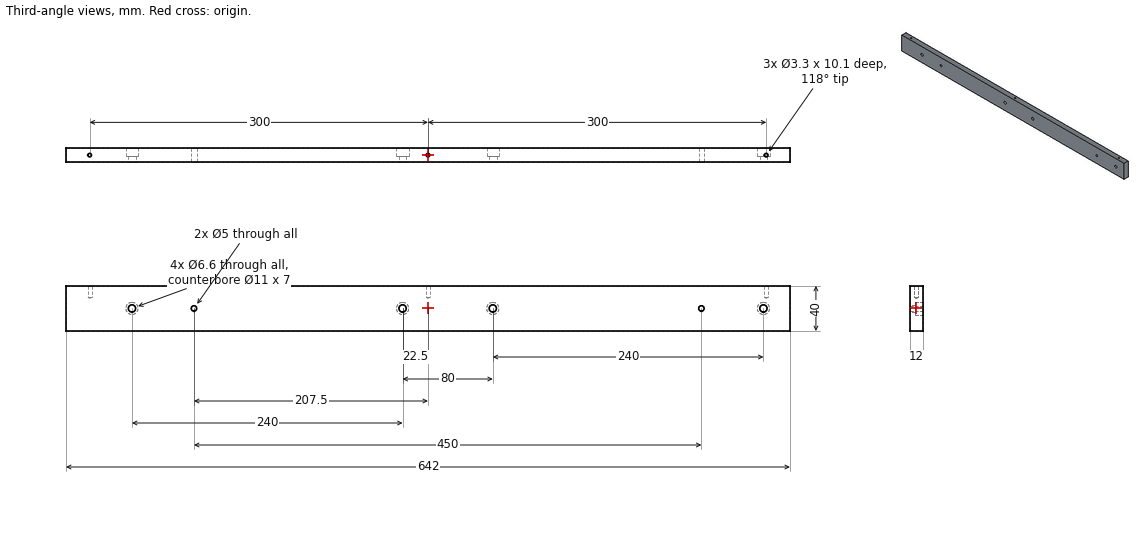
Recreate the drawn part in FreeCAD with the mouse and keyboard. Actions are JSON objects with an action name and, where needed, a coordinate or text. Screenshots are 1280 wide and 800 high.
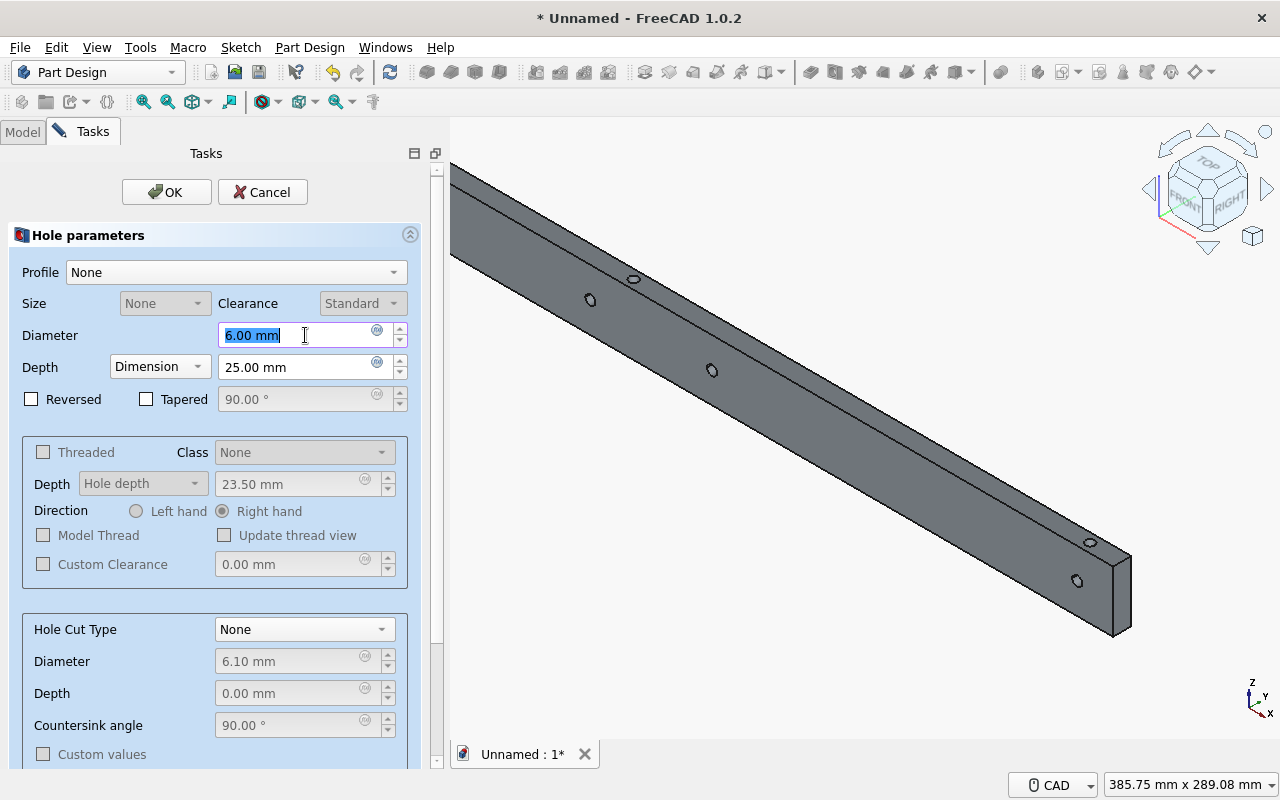
{"action": "type", "text": "3.3"}
{"action": "key", "text": "Tab"}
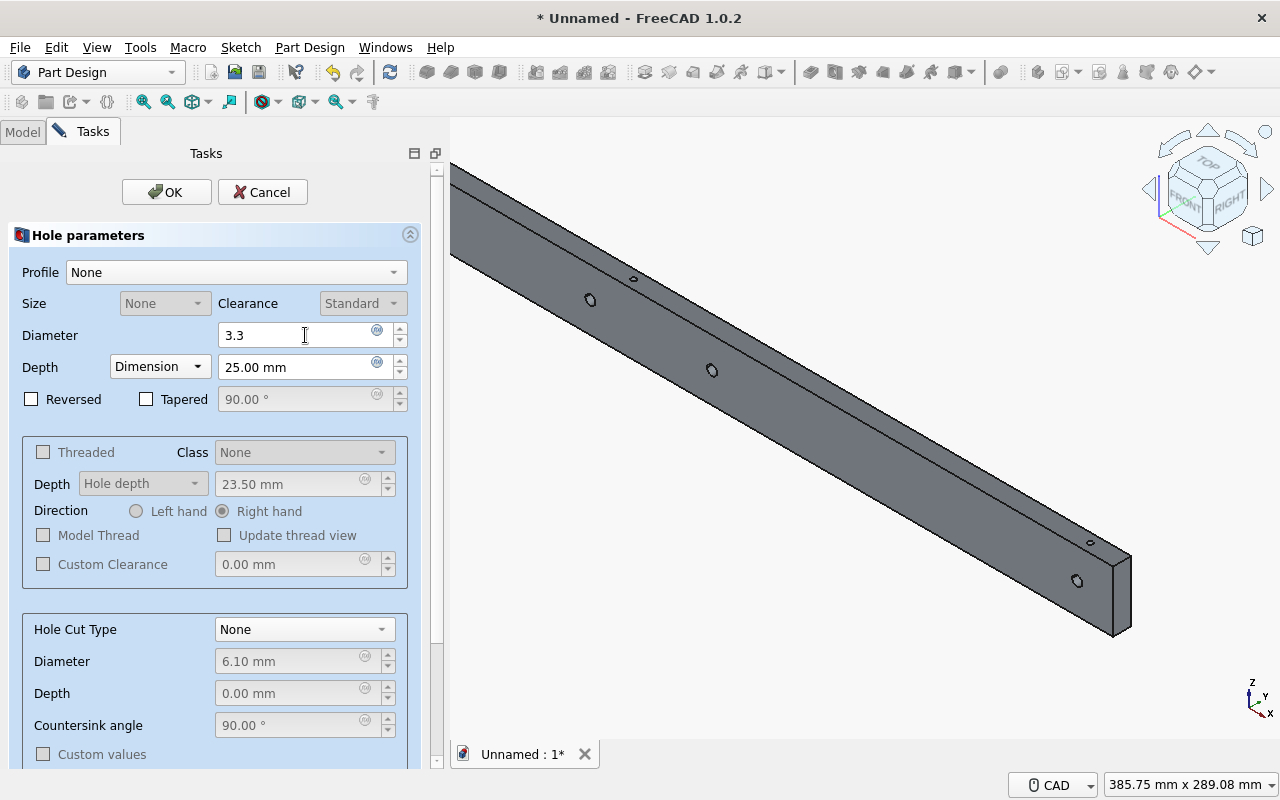
{"action": "triple_click", "coordinate": [305, 367]}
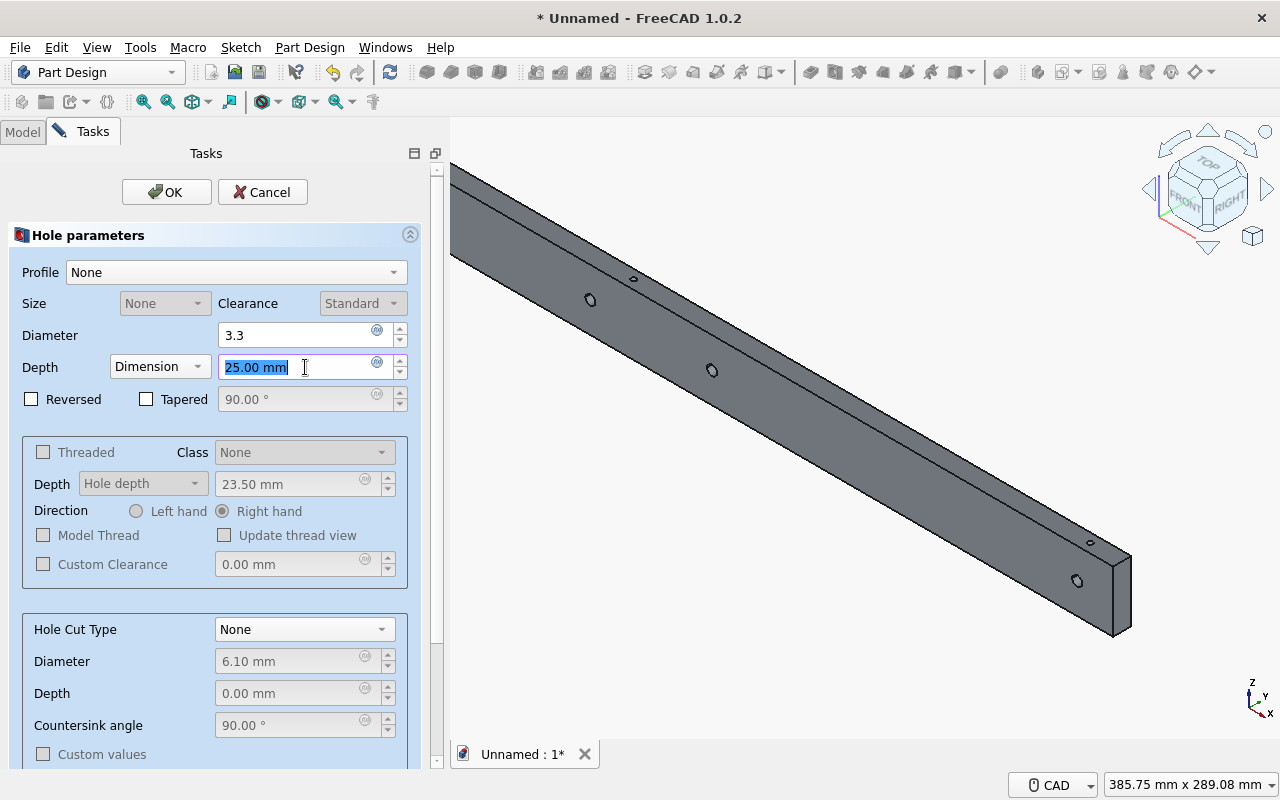
{"action": "type", "text": "10.1"}
{"action": "key", "text": "Tab"}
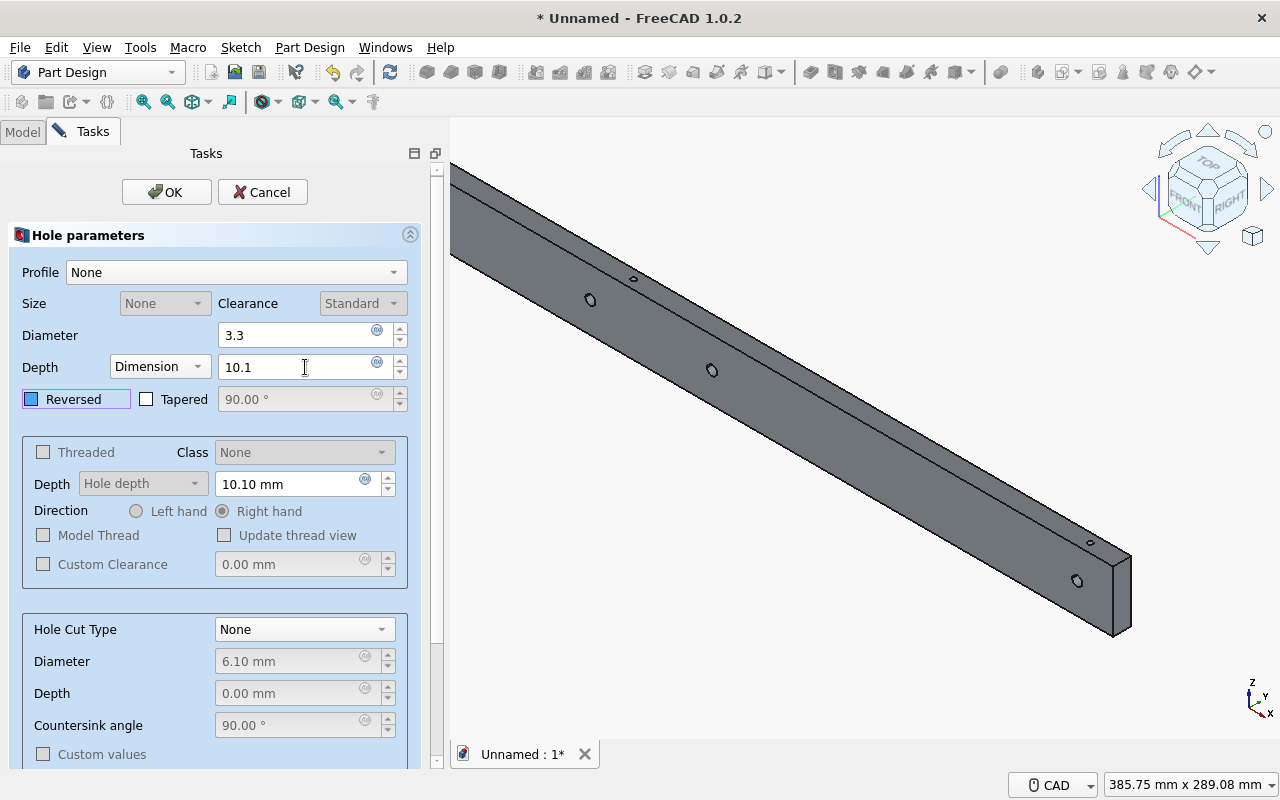
{"action": "left_click", "coordinate": [167, 192]}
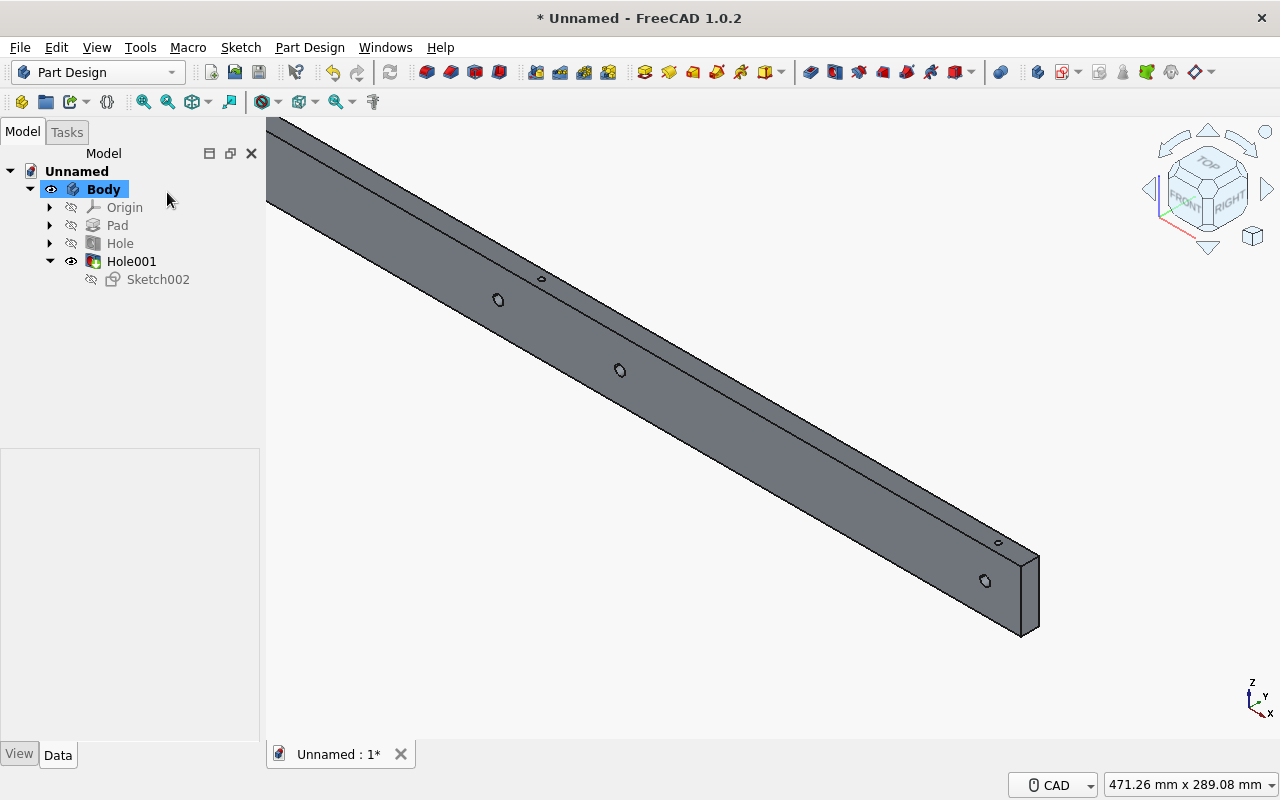
{"action": "left_click", "coordinate": [144, 102]}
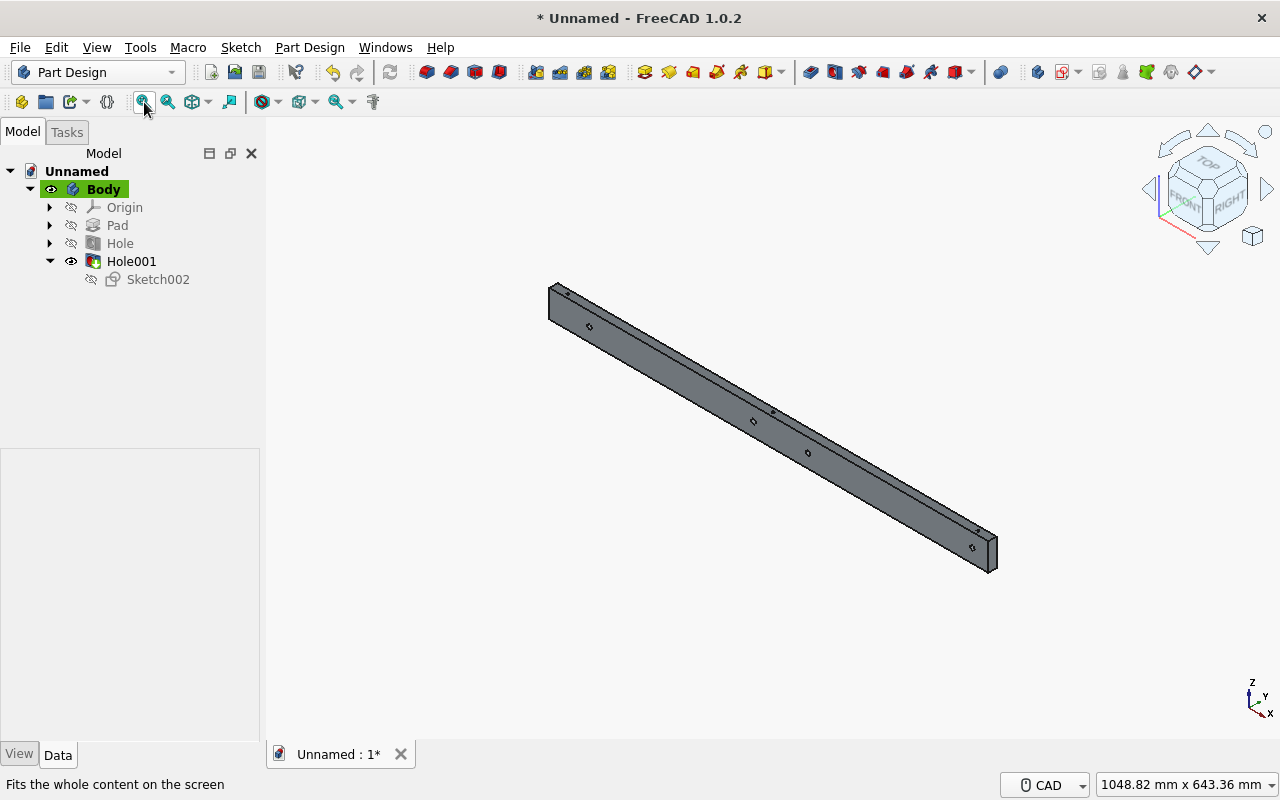
{"action": "key", "text": "4"}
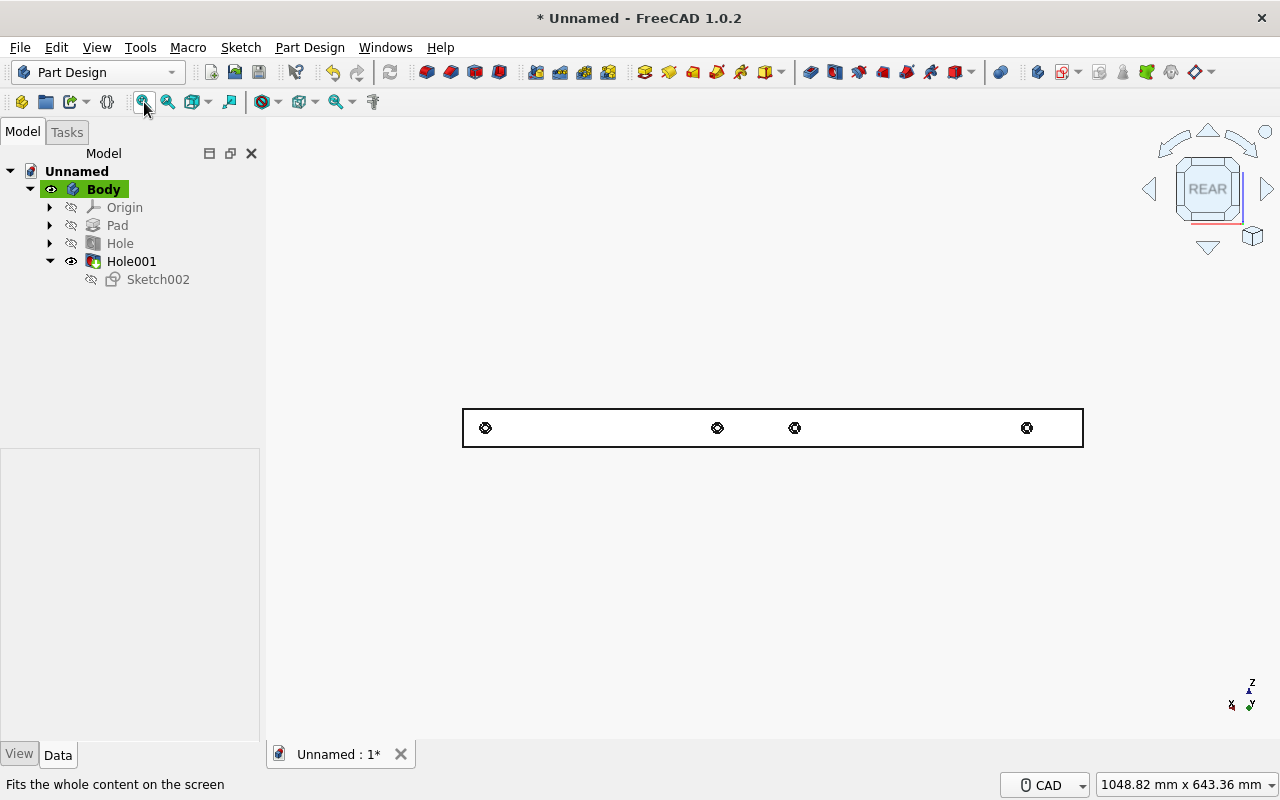
{"action": "left_click", "coordinate": [596, 427]}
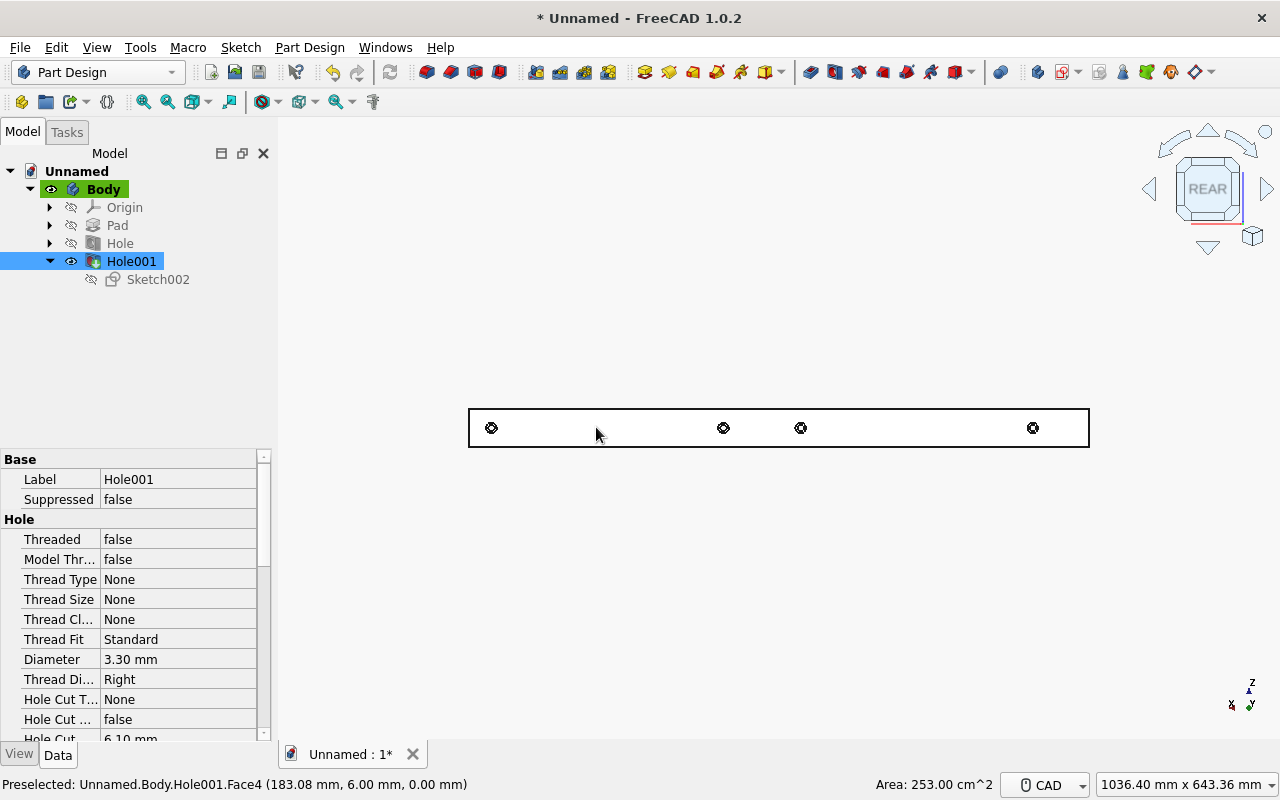
{"action": "left_click", "coordinate": [1062, 72]}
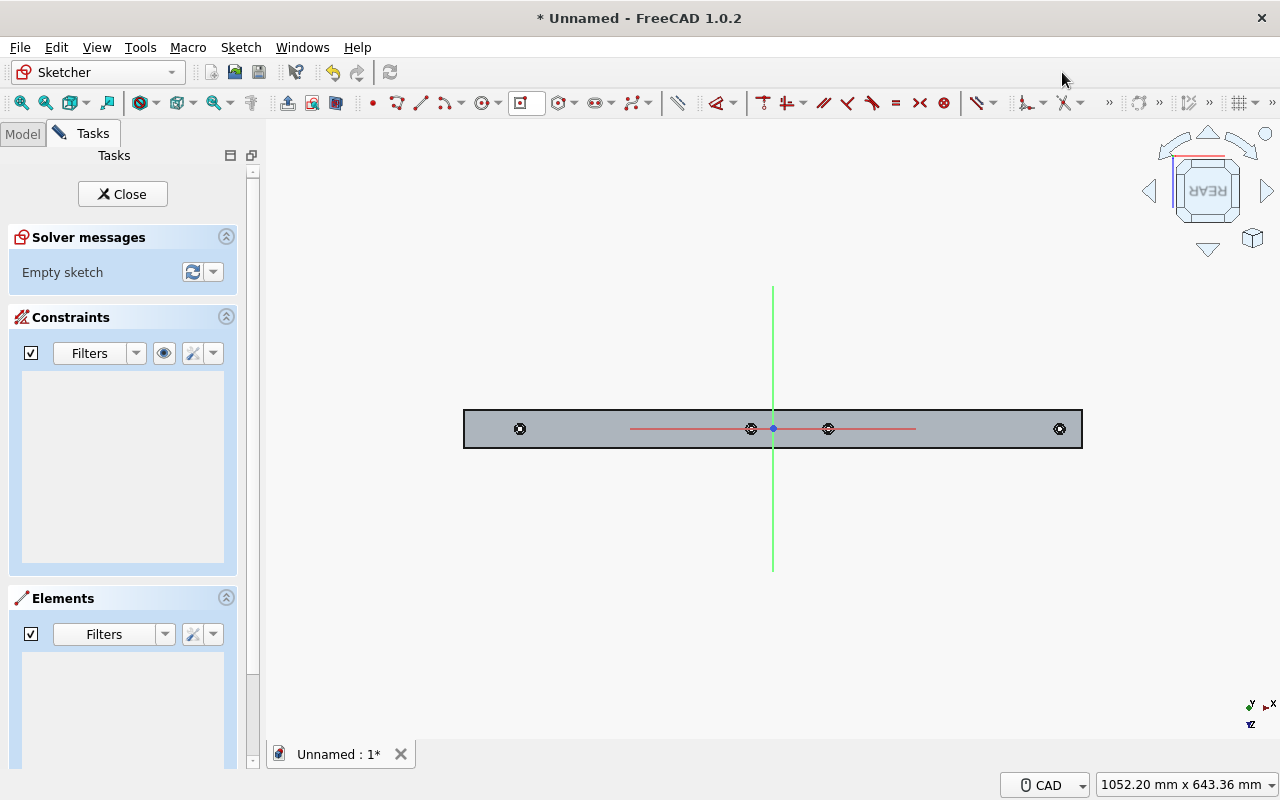
{"action": "left_click", "coordinate": [482, 104]}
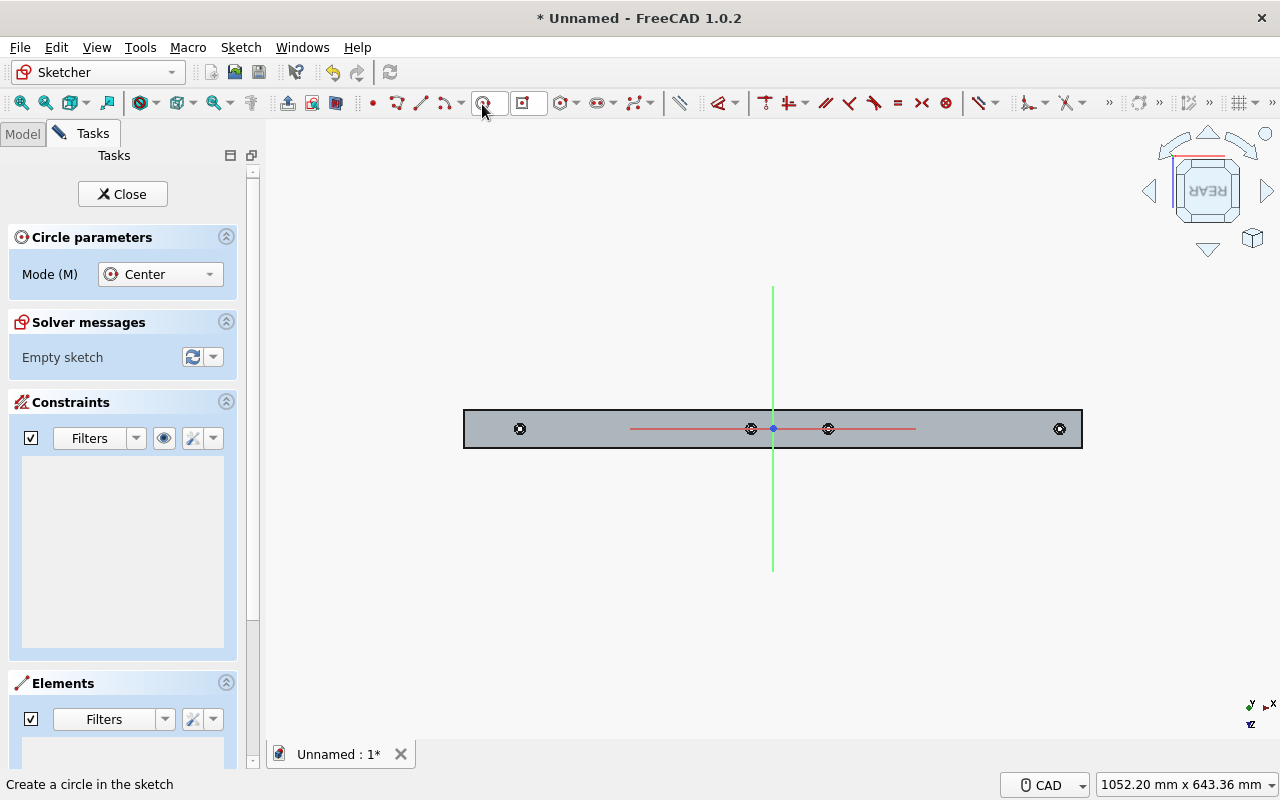
{"action": "scroll", "coordinate": [573, 429], "scroll_direction": "up", "scroll_amount": 12}